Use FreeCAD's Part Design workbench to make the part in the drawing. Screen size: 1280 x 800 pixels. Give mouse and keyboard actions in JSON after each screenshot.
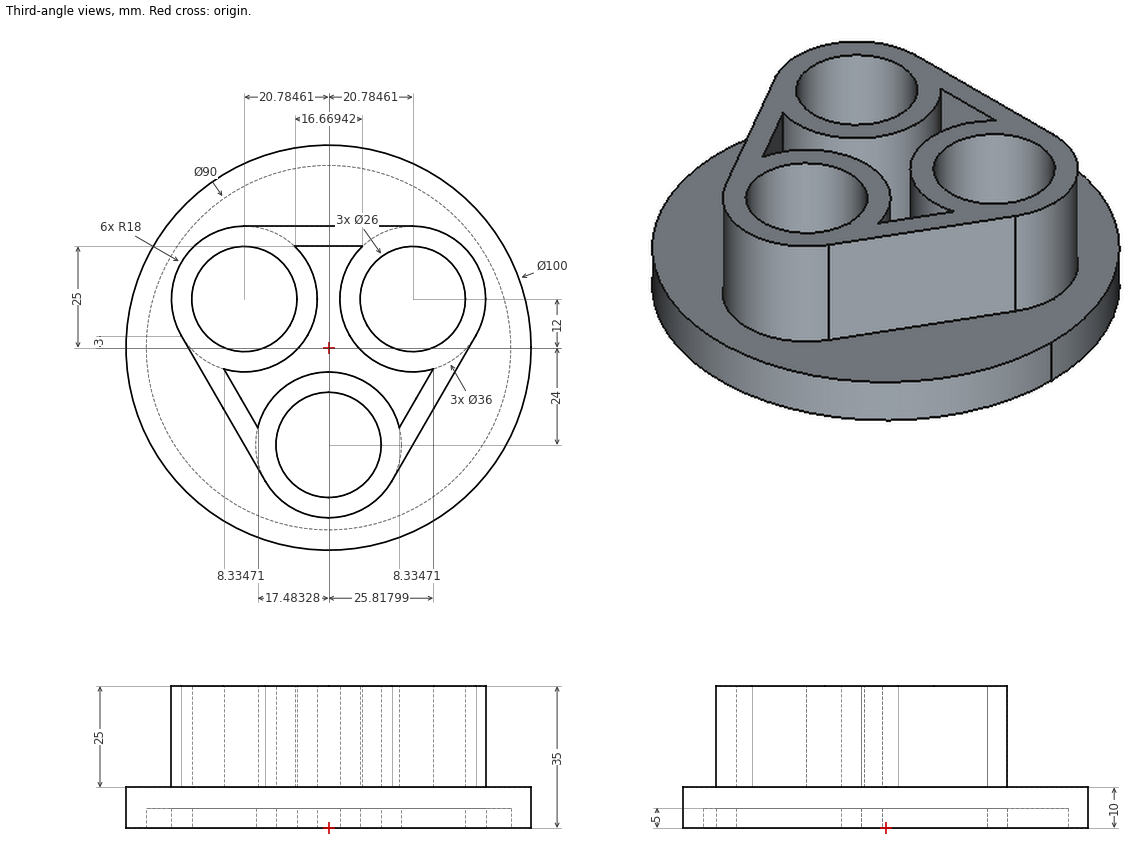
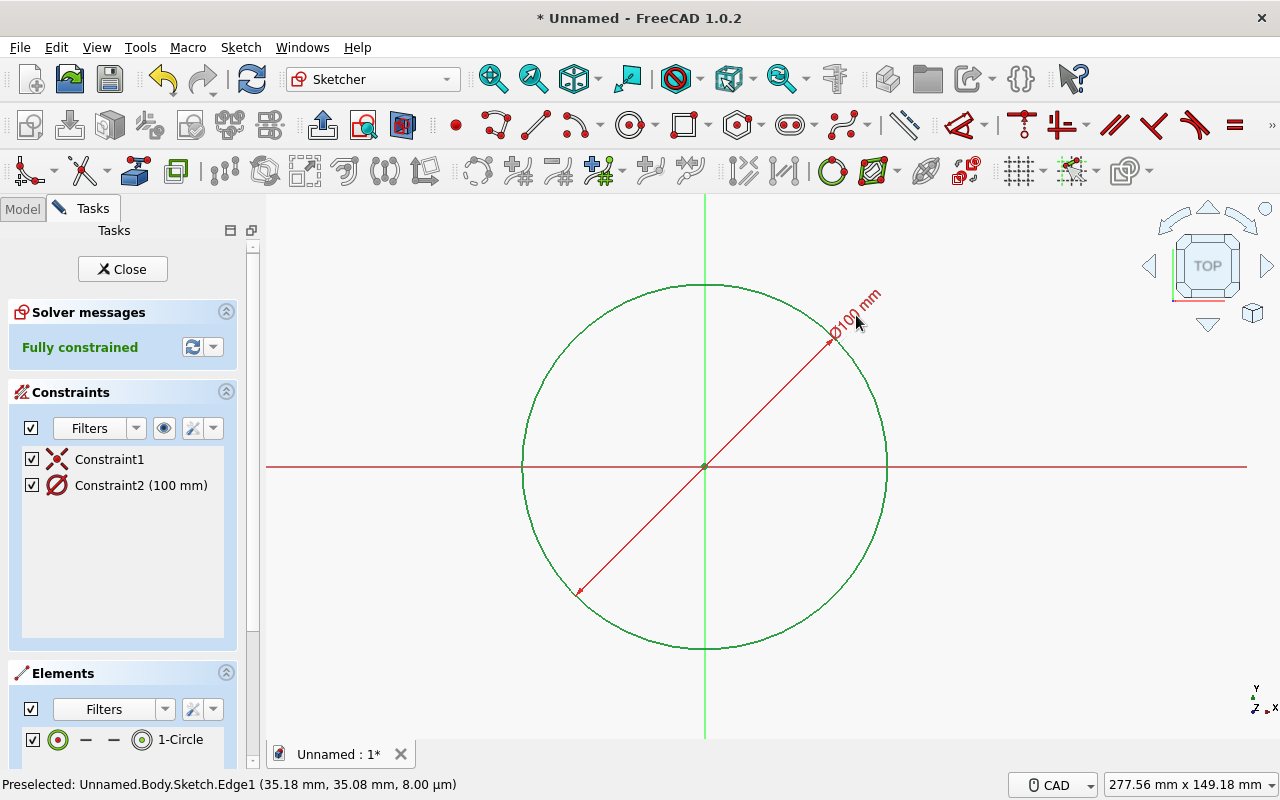
{"action": "left_click", "coordinate": [123, 269]}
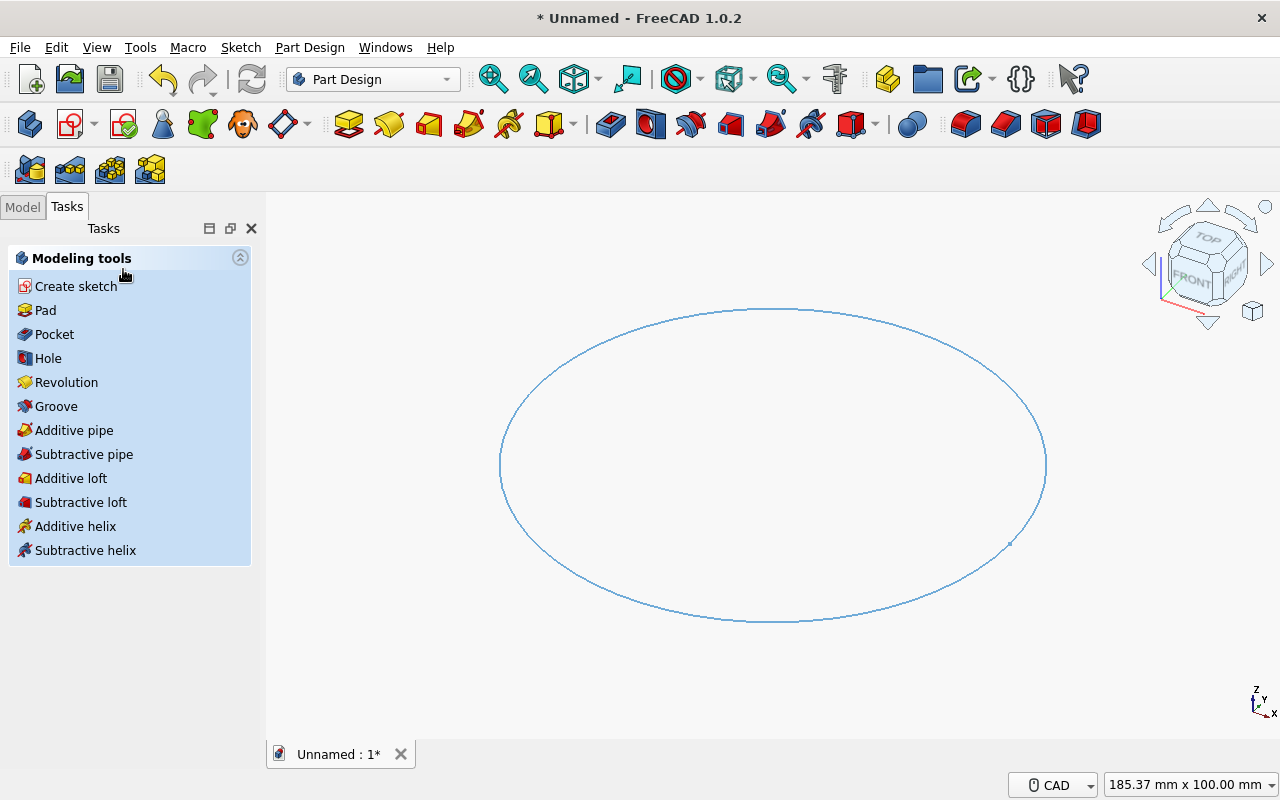
{"action": "left_click", "coordinate": [350, 124]}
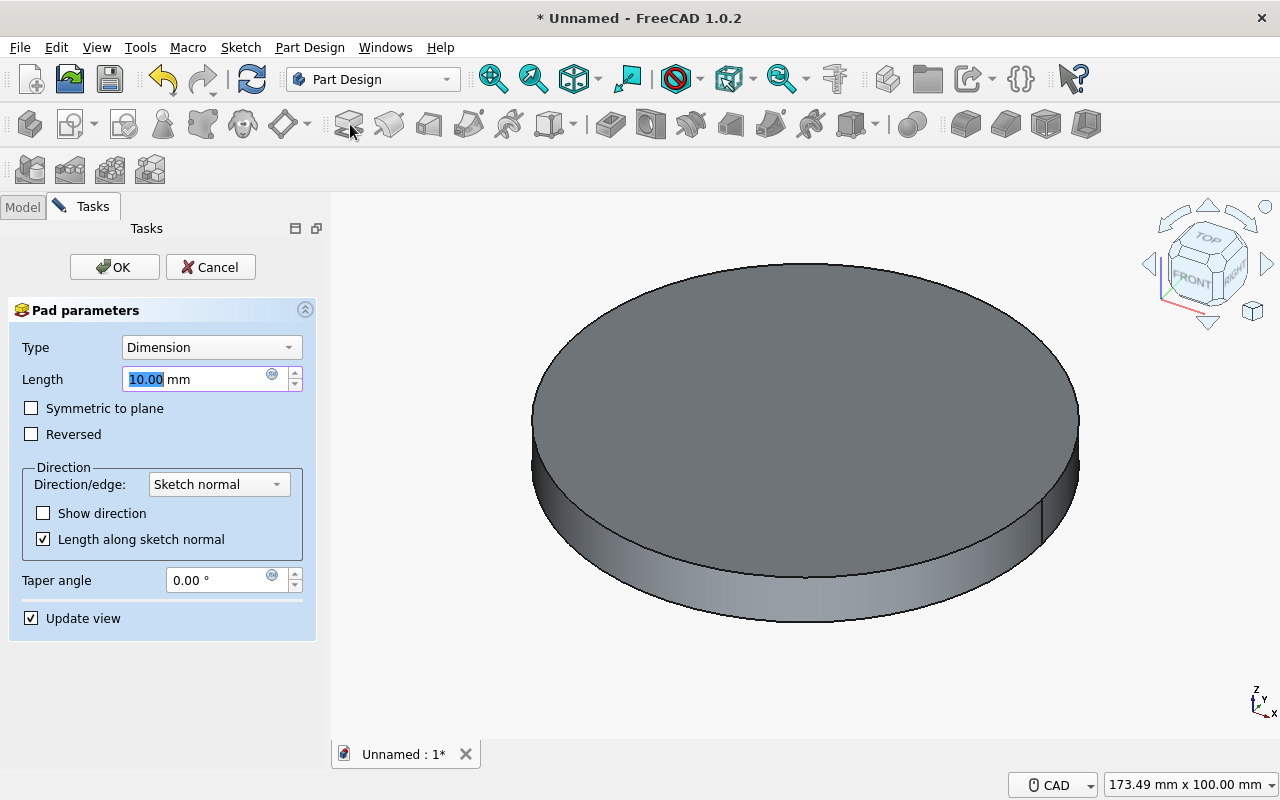
{"action": "type", "text": "10"}
{"action": "key", "text": "Tab"}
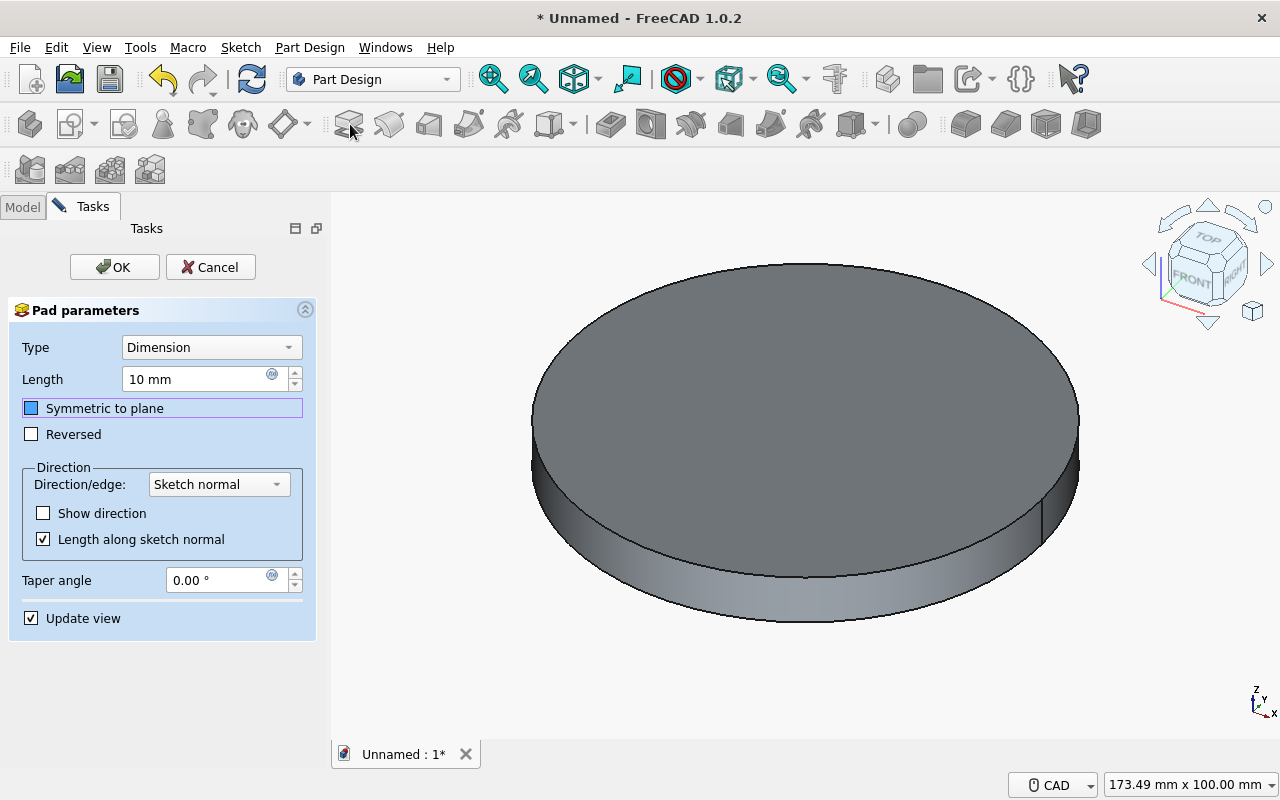
{"action": "left_click", "coordinate": [115, 267]}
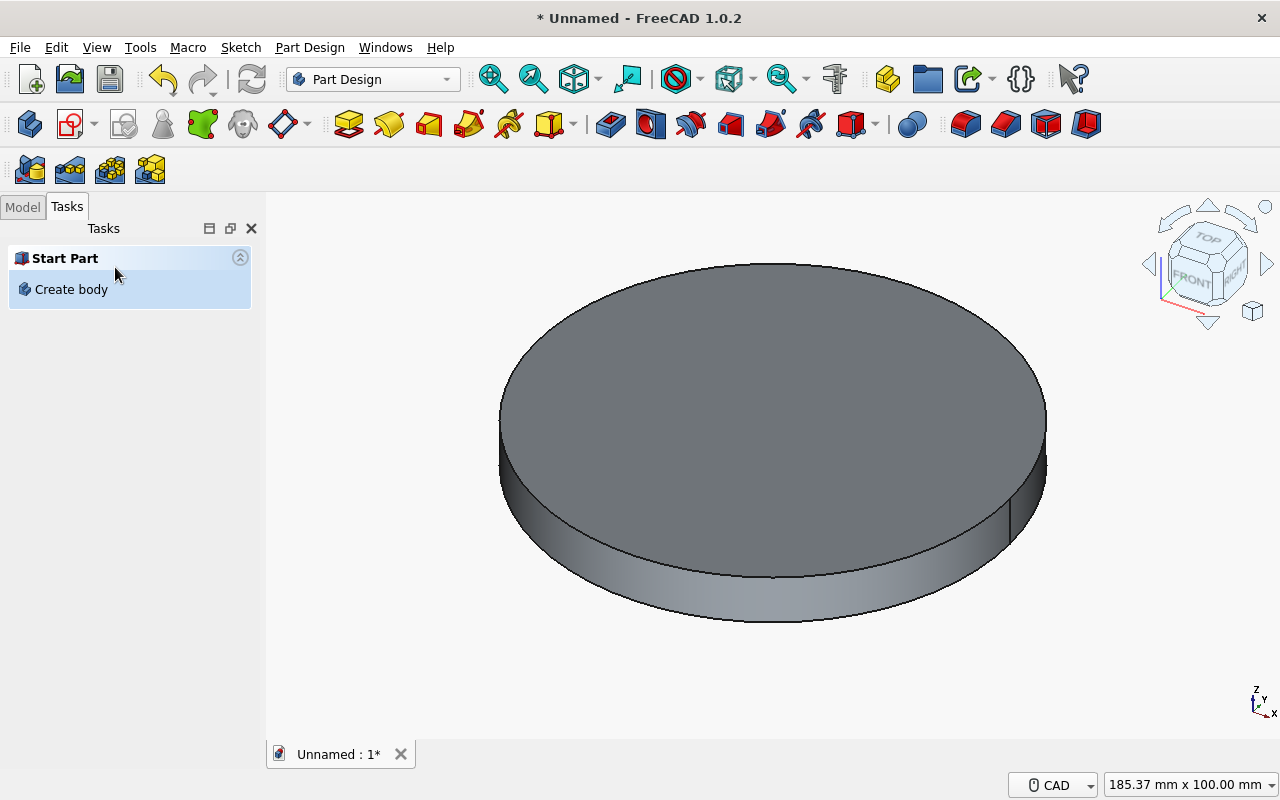
{"action": "left_click", "coordinate": [773, 420]}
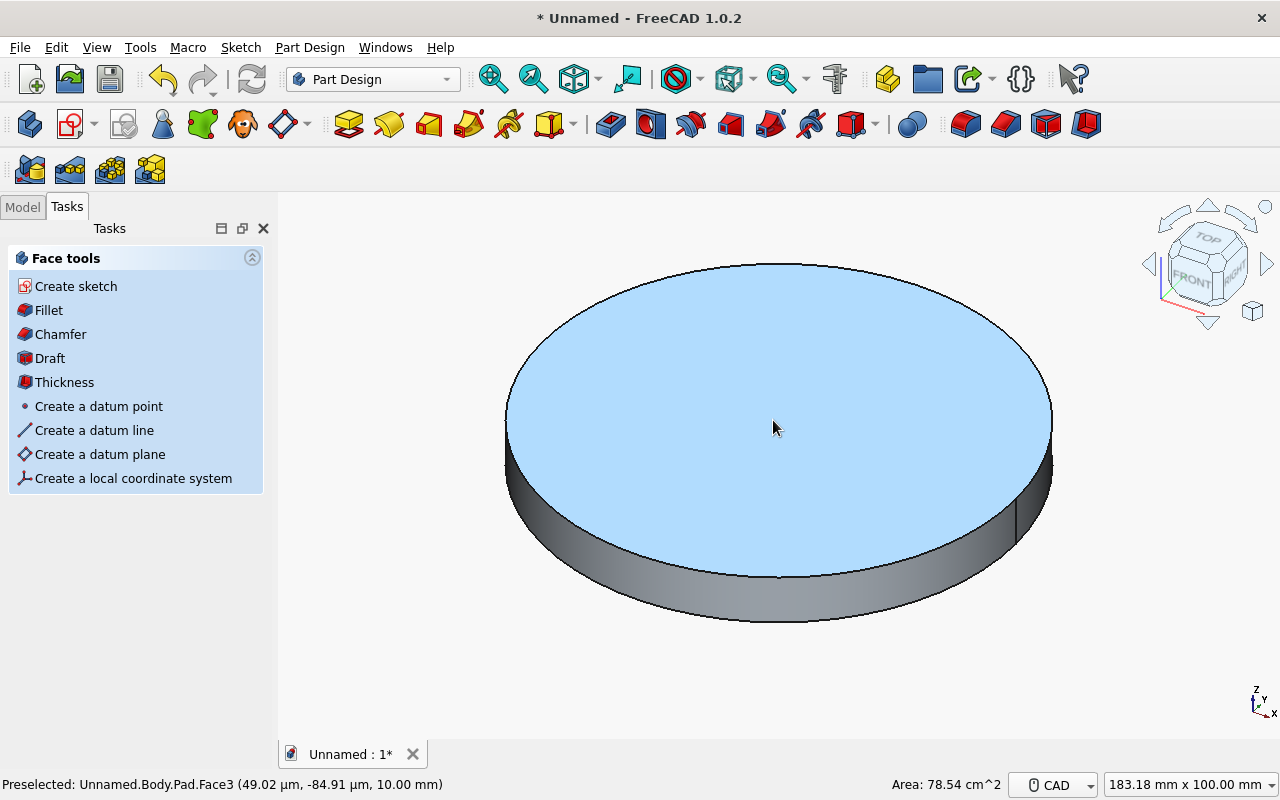
{"action": "left_click", "coordinate": [70, 124]}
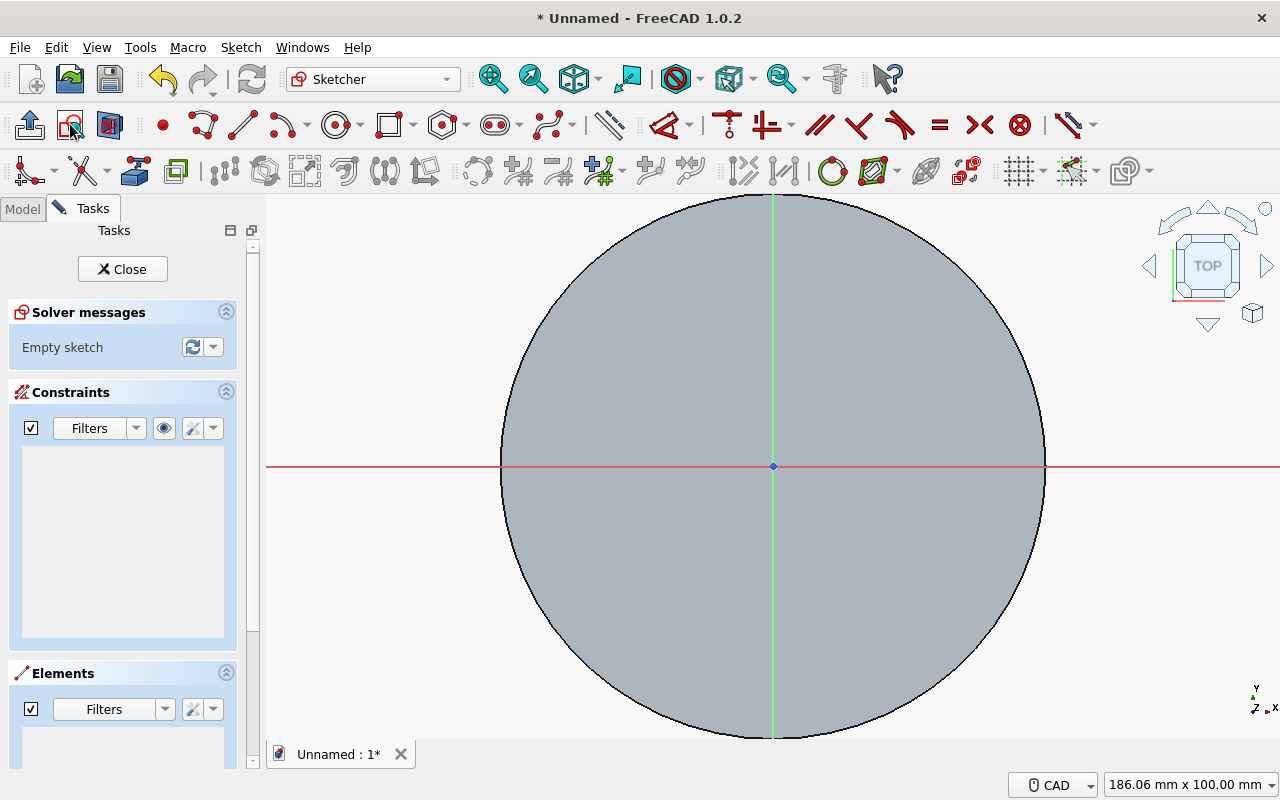
{"action": "scroll", "coordinate": [395, 319], "scroll_direction": "down", "scroll_amount": 1}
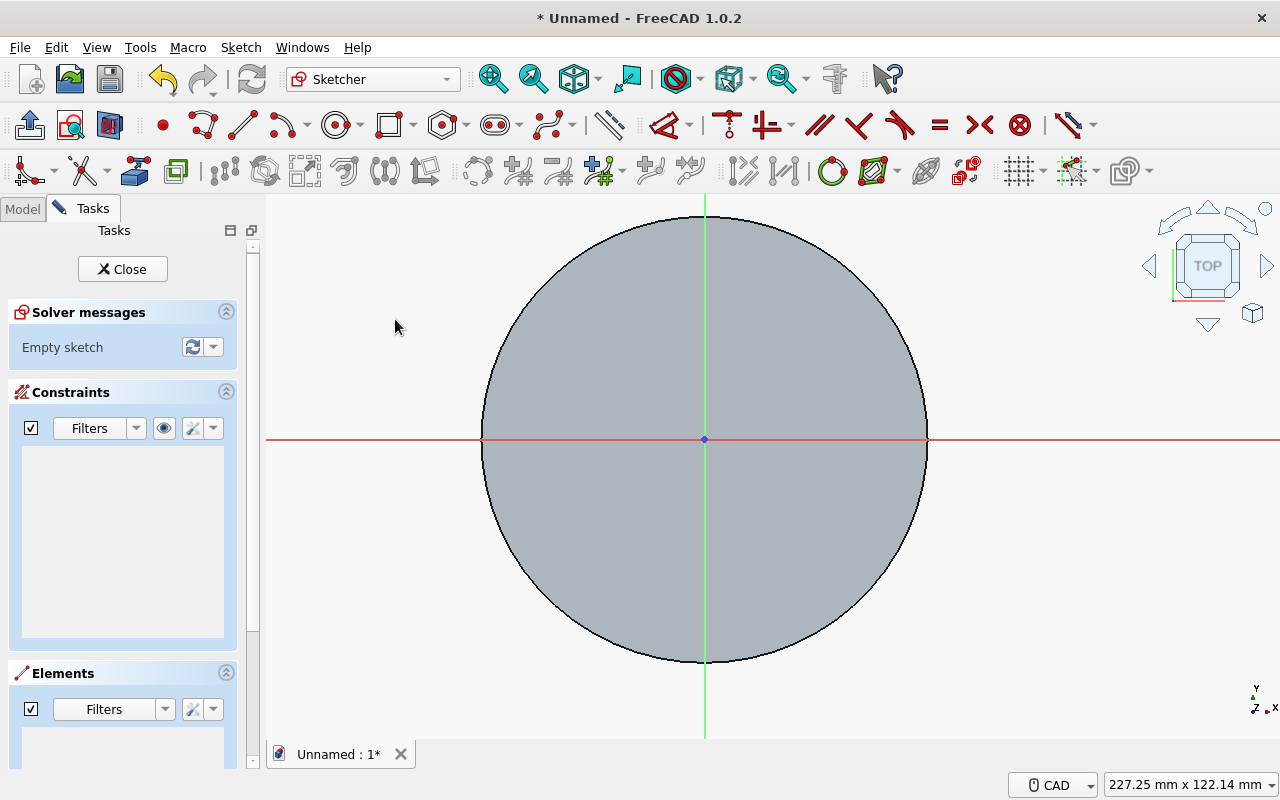
{"action": "left_click", "coordinate": [244, 126]}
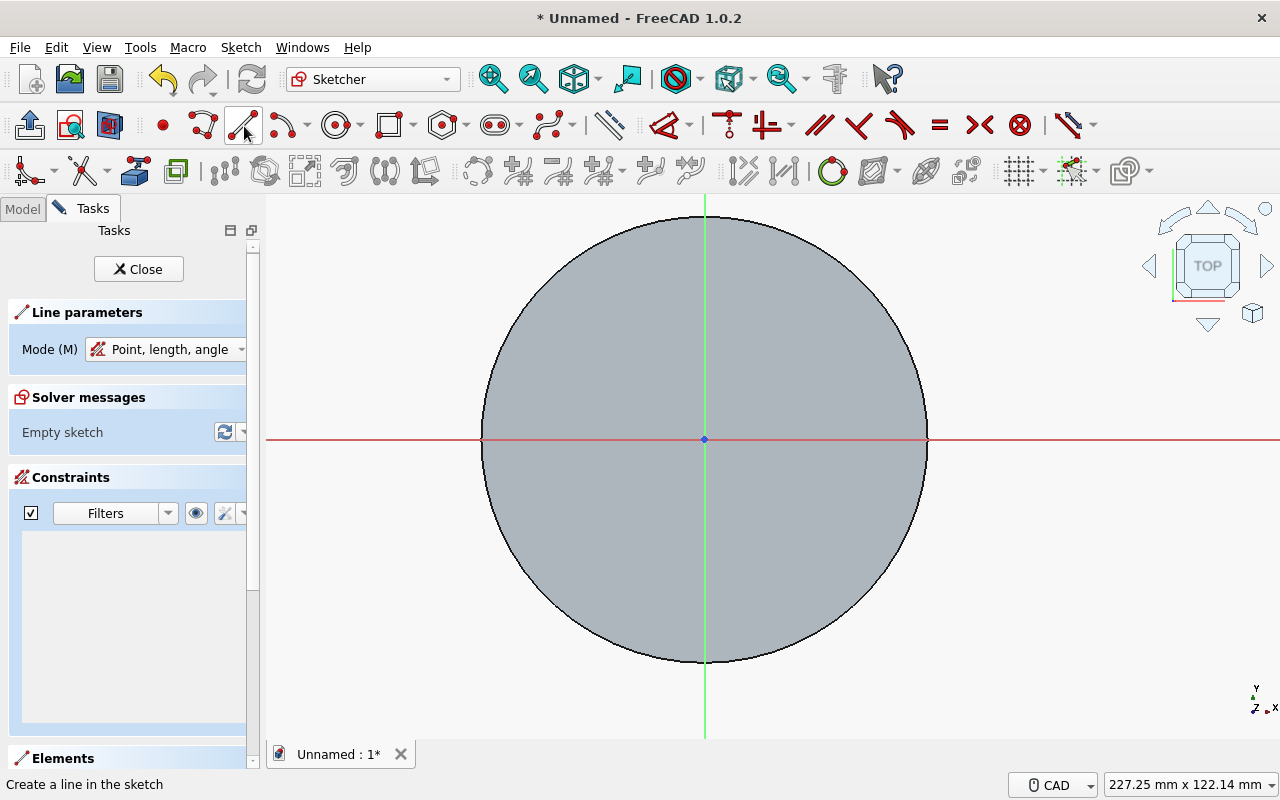
{"action": "left_click", "coordinate": [542, 426]}
{"action": "left_click", "coordinate": [635, 587]}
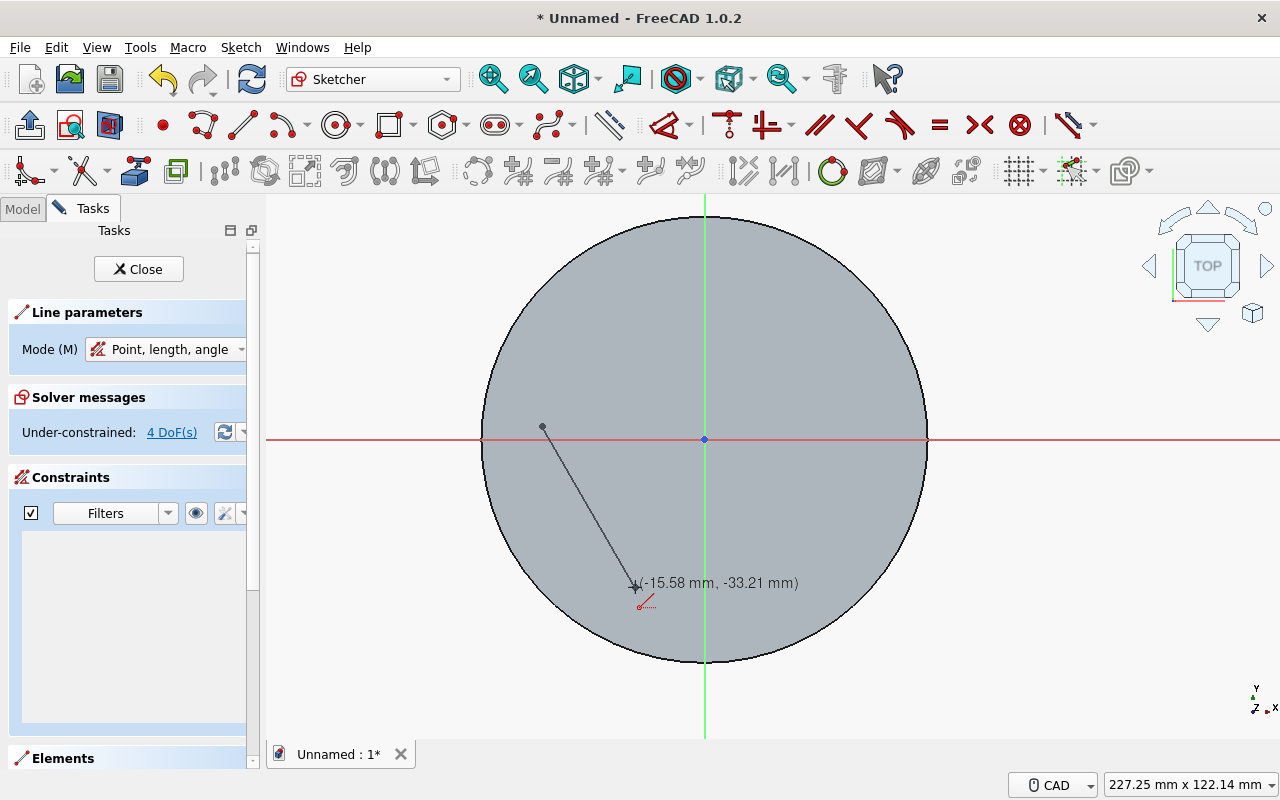
{"action": "left_click", "coordinate": [774, 587]}
{"action": "left_click", "coordinate": [867, 426]}